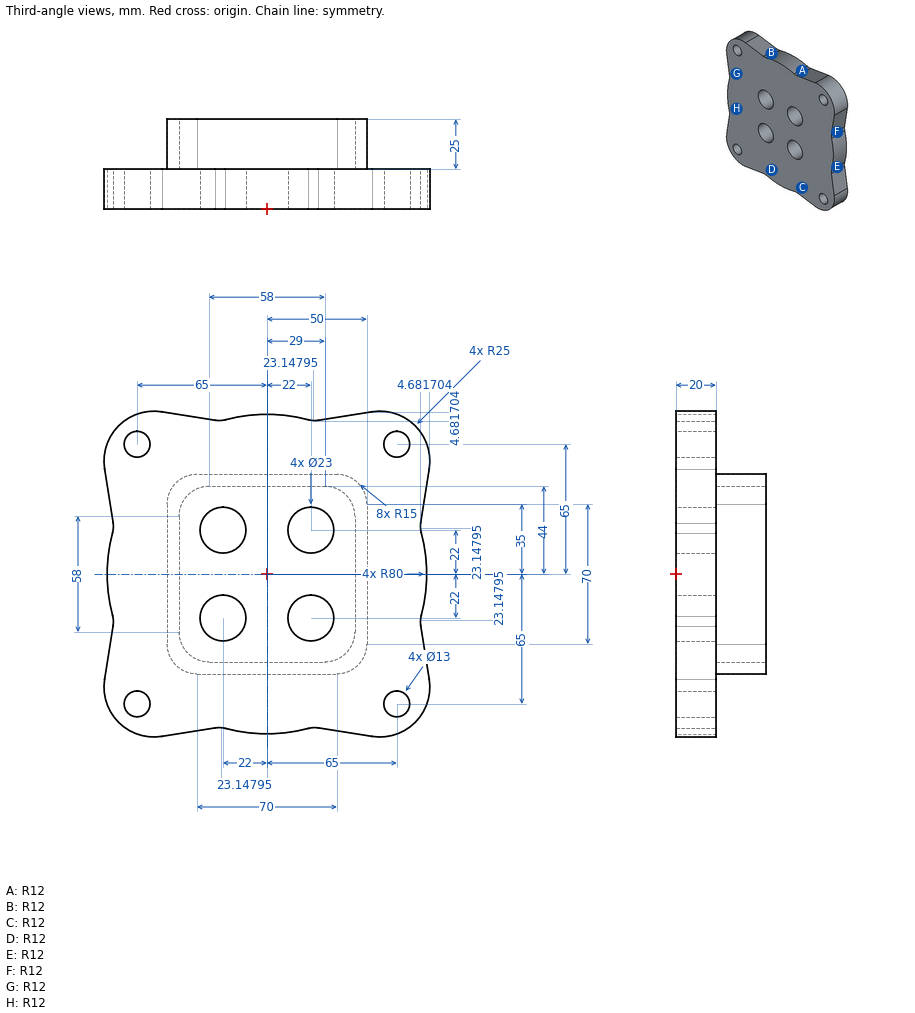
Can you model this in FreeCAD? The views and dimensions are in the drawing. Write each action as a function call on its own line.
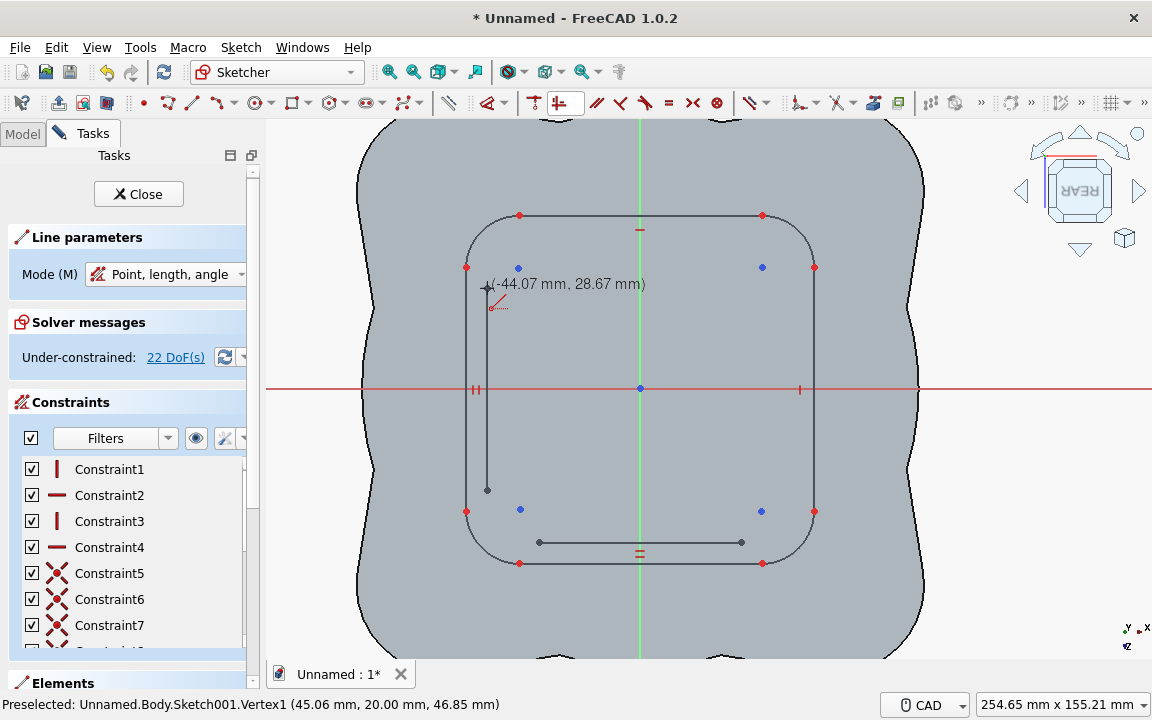
click(539, 236)
click(741, 236)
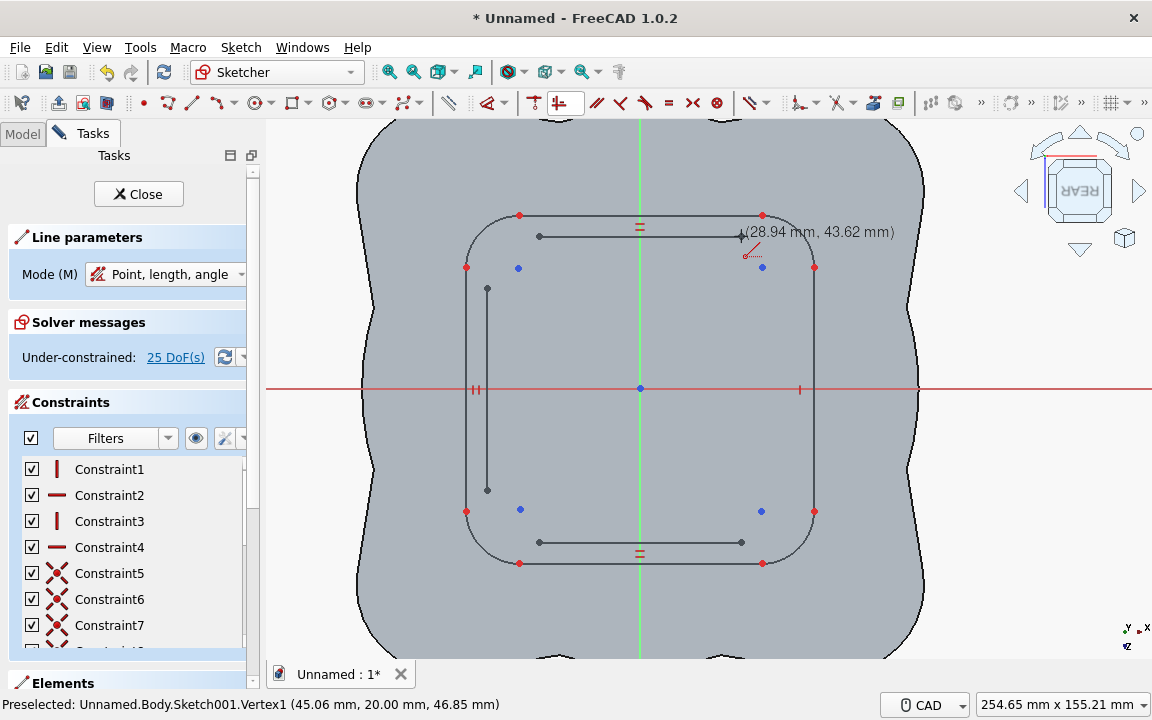
click(793, 288)
click(793, 490)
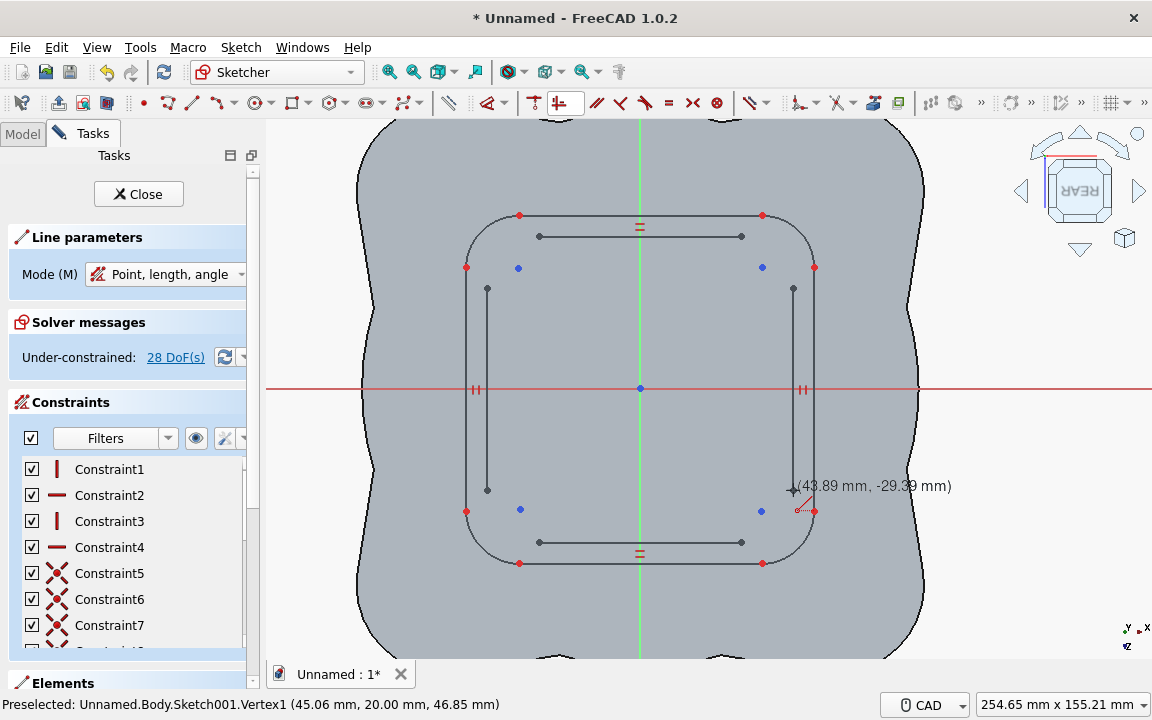
click(218, 104)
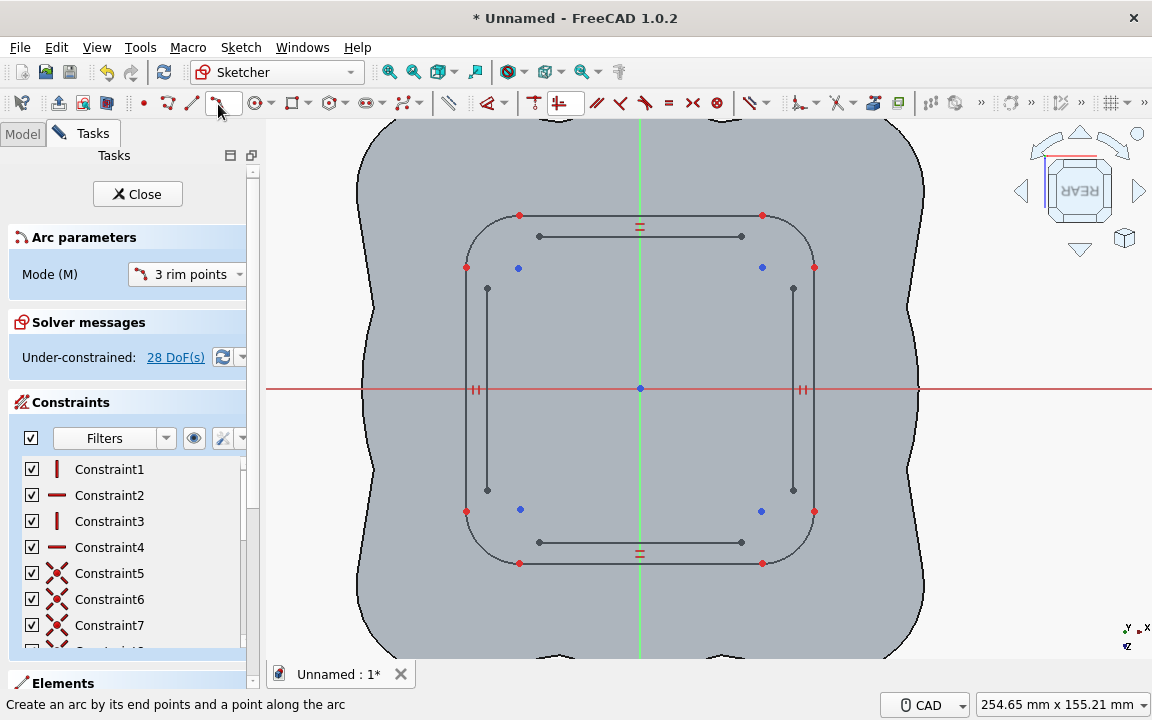
click(539, 543)
click(487, 491)
click(503, 527)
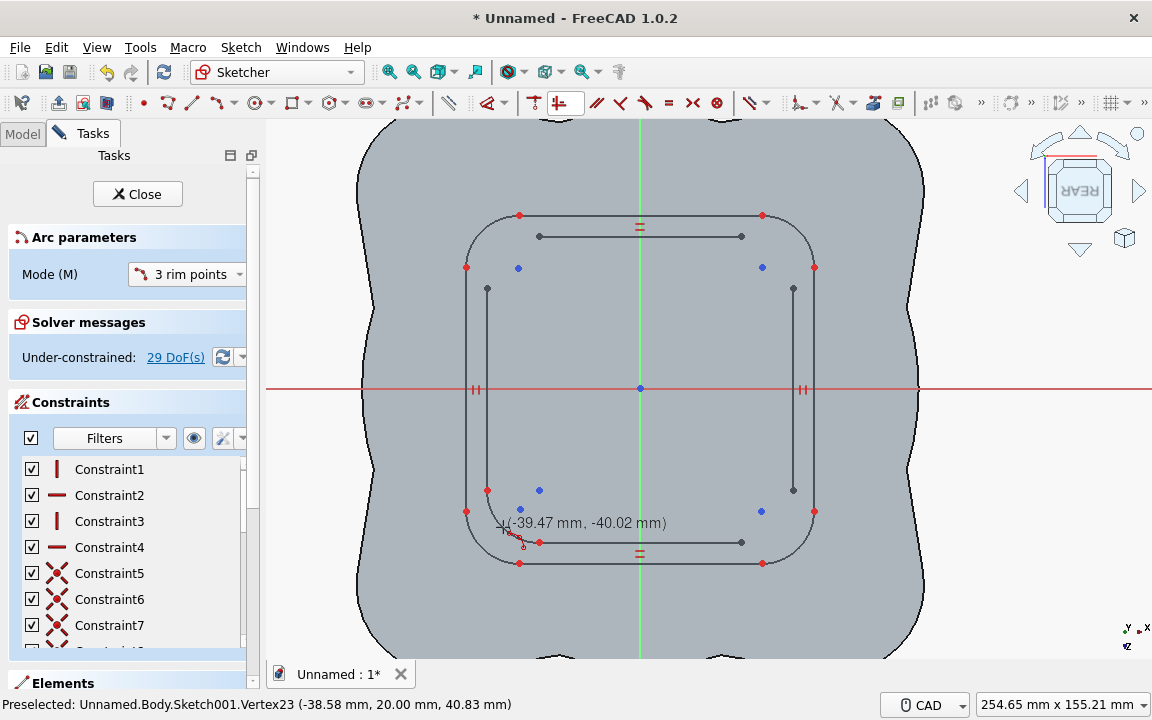
click(487, 289)
click(539, 237)
click(503, 251)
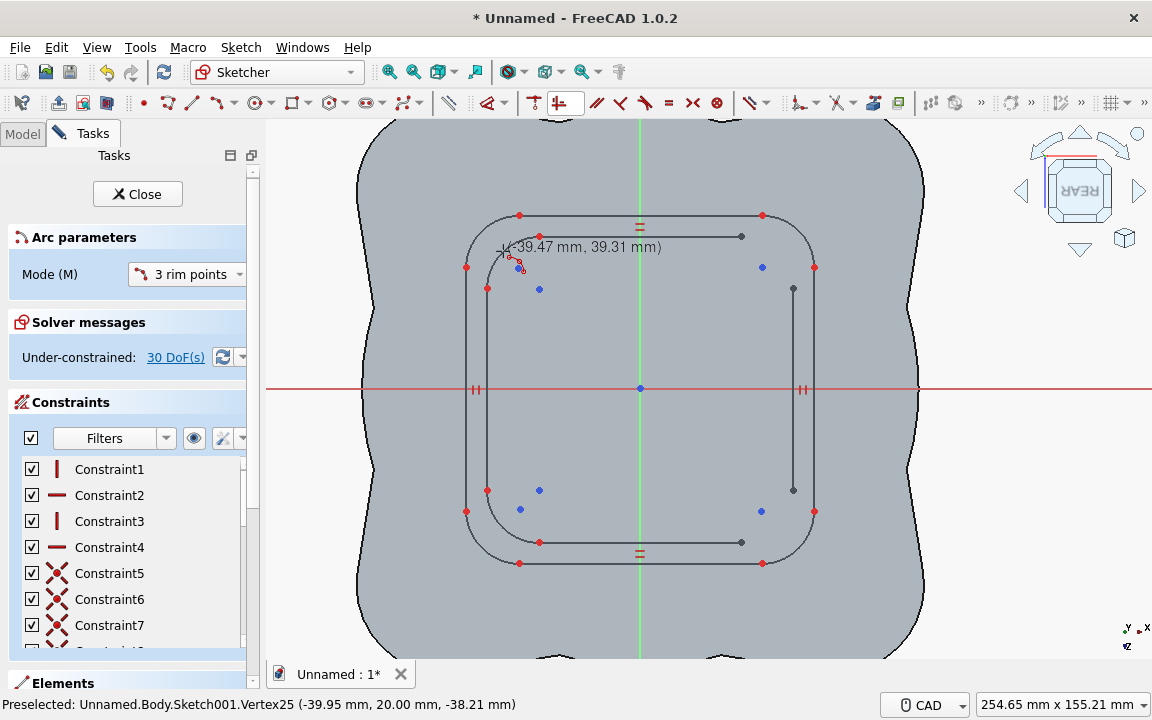
click(741, 237)
click(793, 289)
click(778, 251)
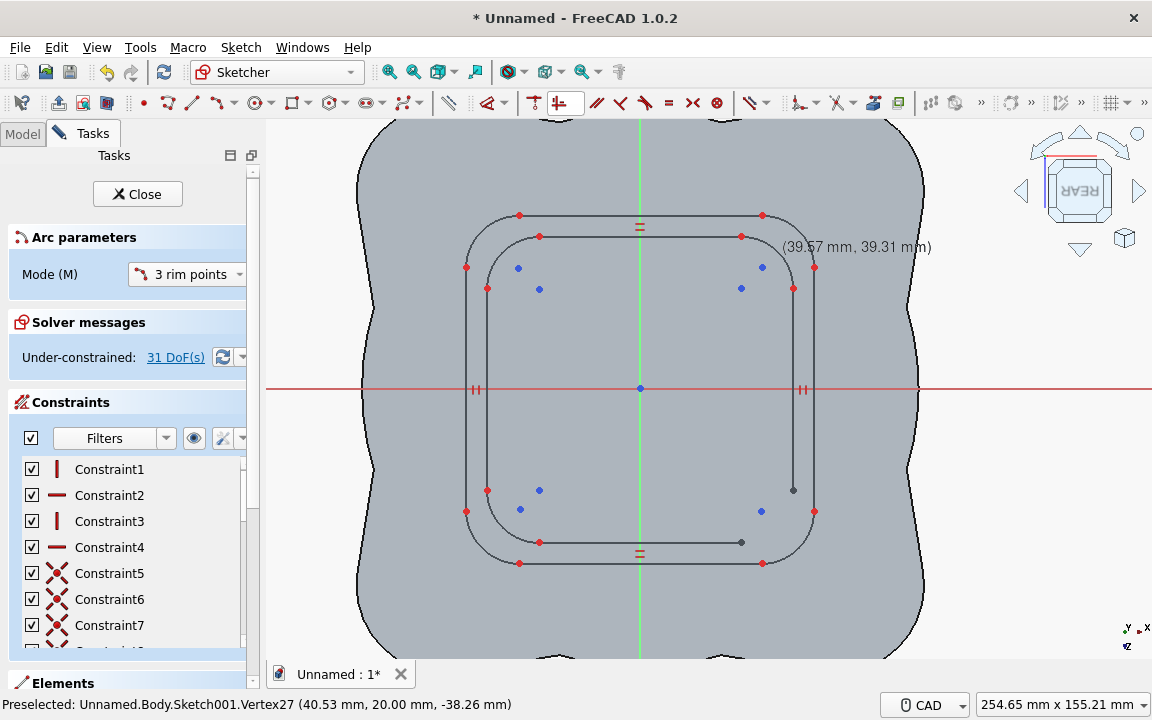
click(793, 491)
click(741, 543)
click(778, 527)
key(Escape)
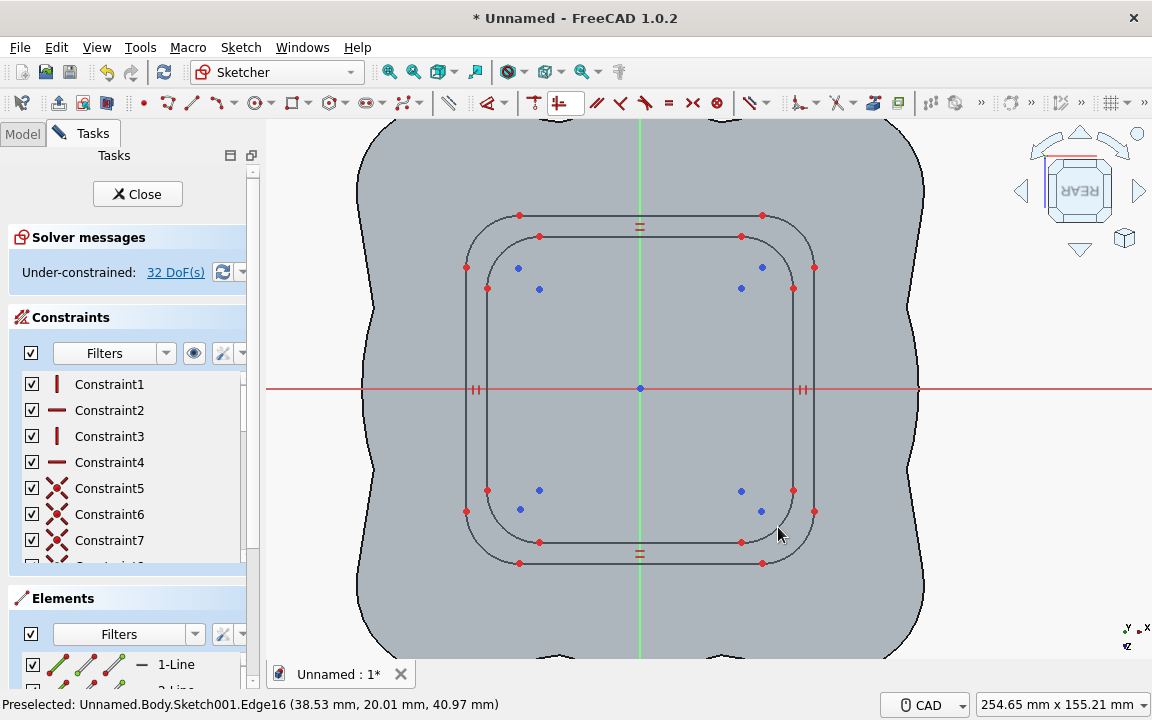
click(814, 439)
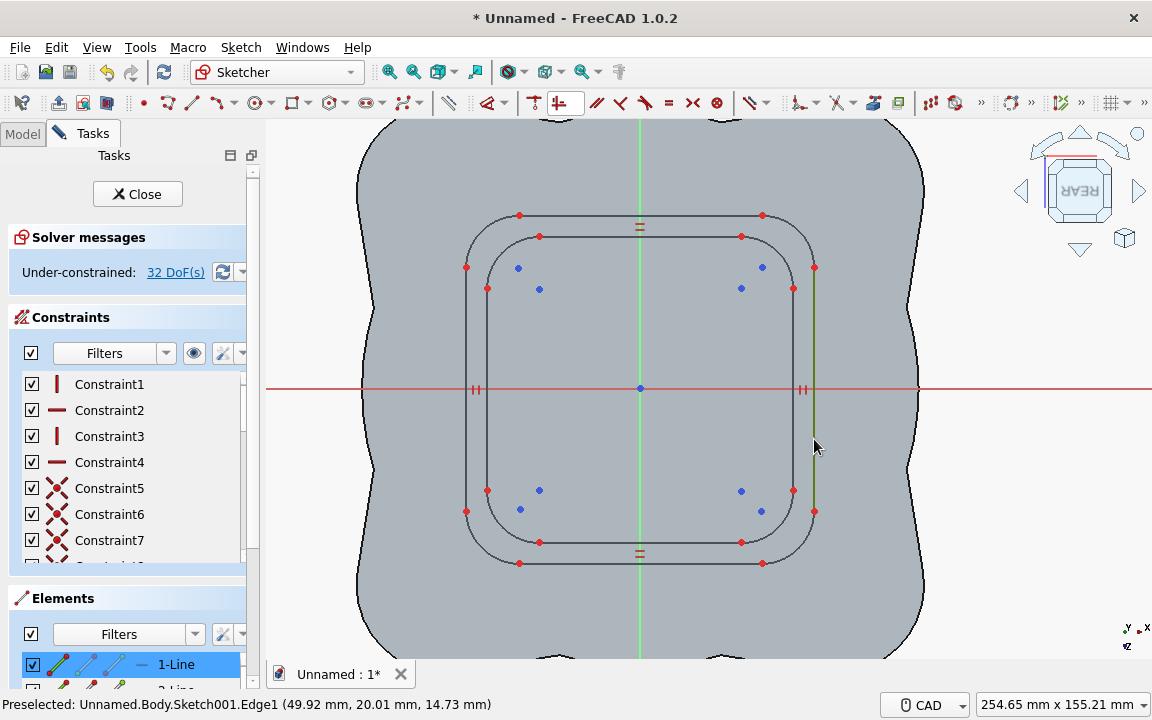
click(809, 244)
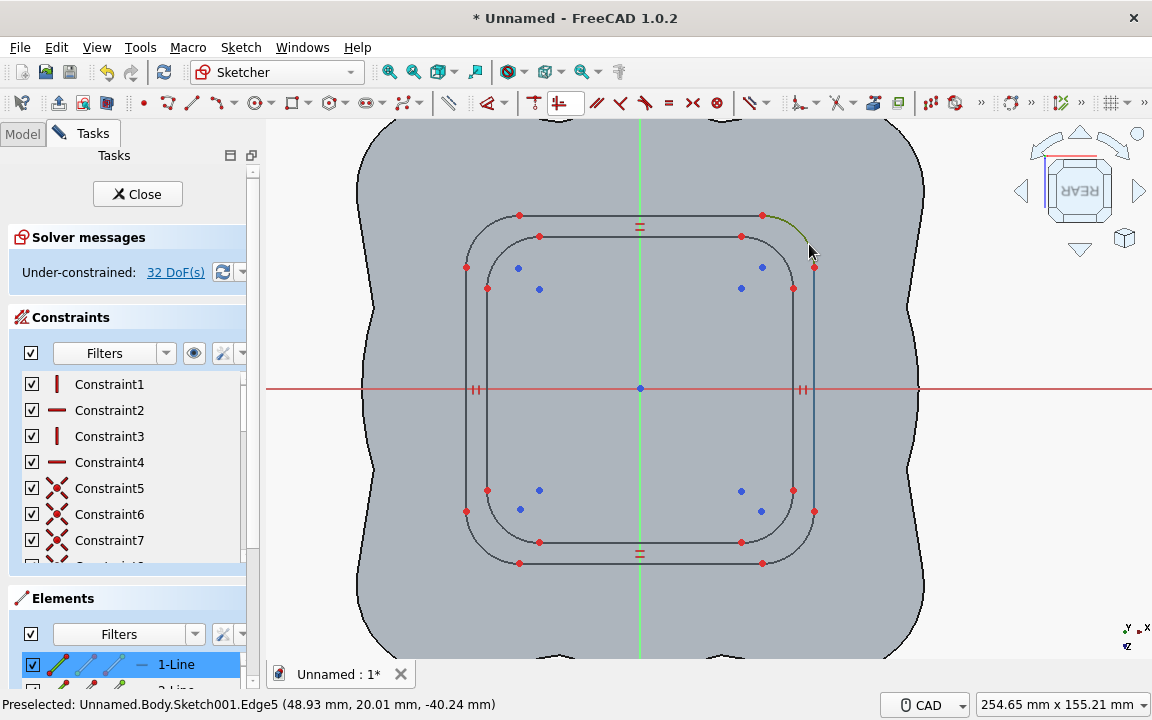
click(646, 104)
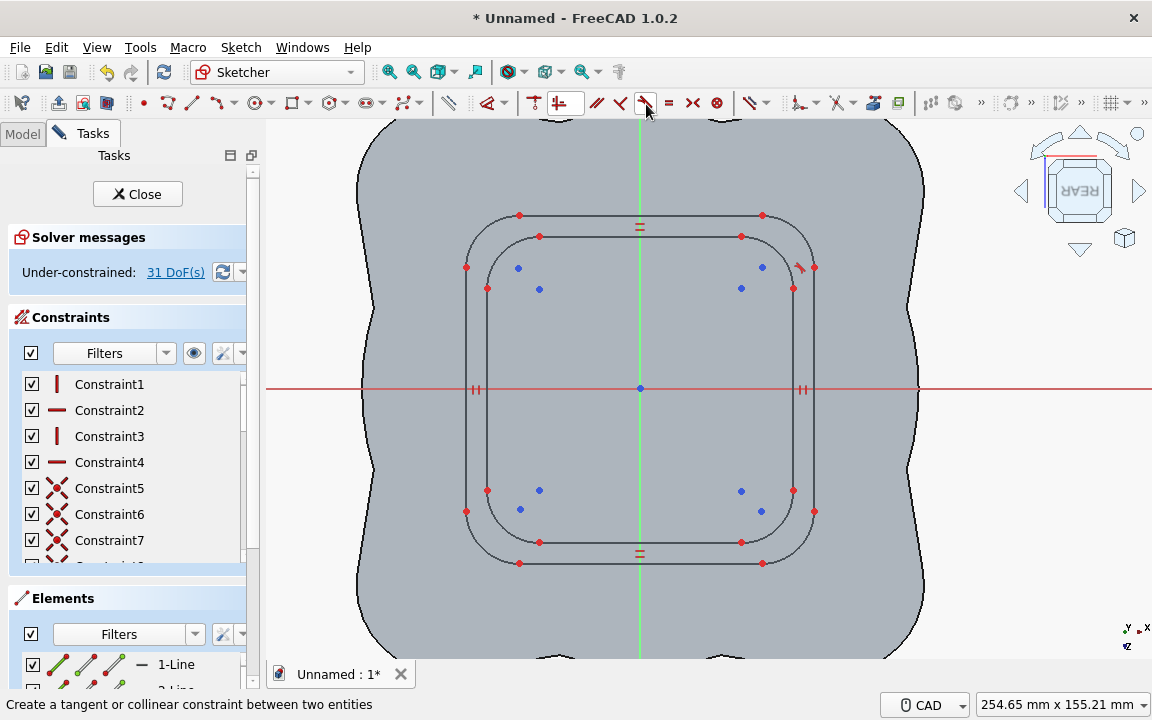
click(814, 439)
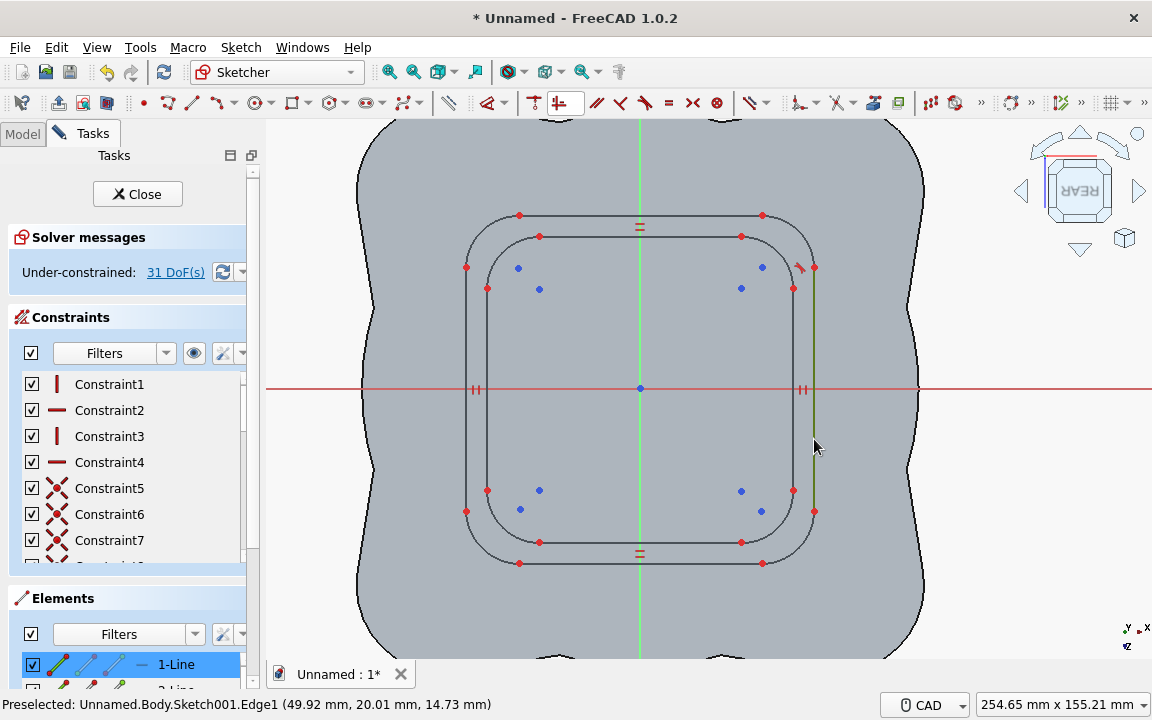
click(785, 558)